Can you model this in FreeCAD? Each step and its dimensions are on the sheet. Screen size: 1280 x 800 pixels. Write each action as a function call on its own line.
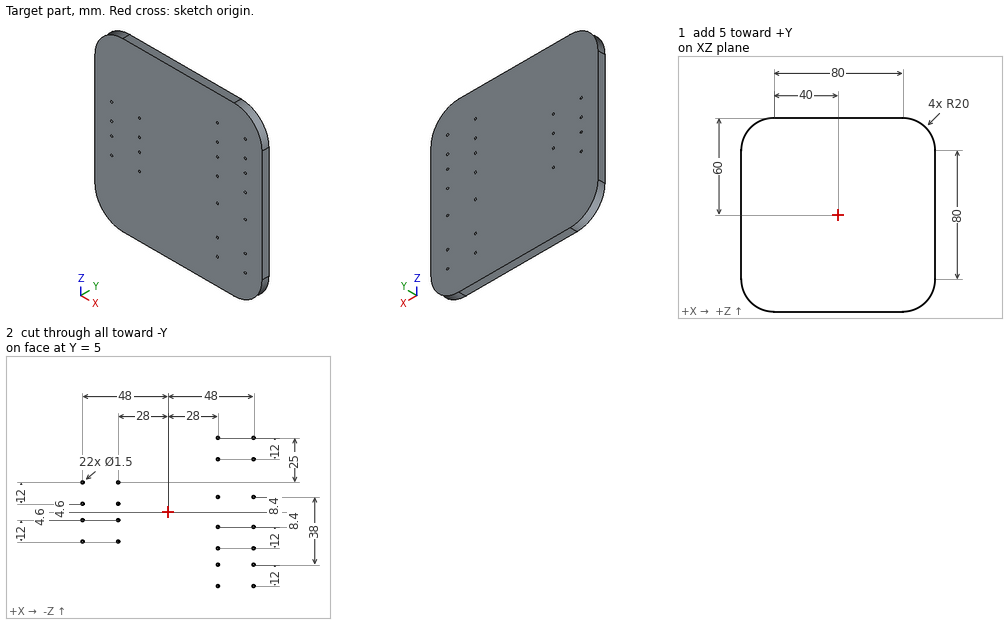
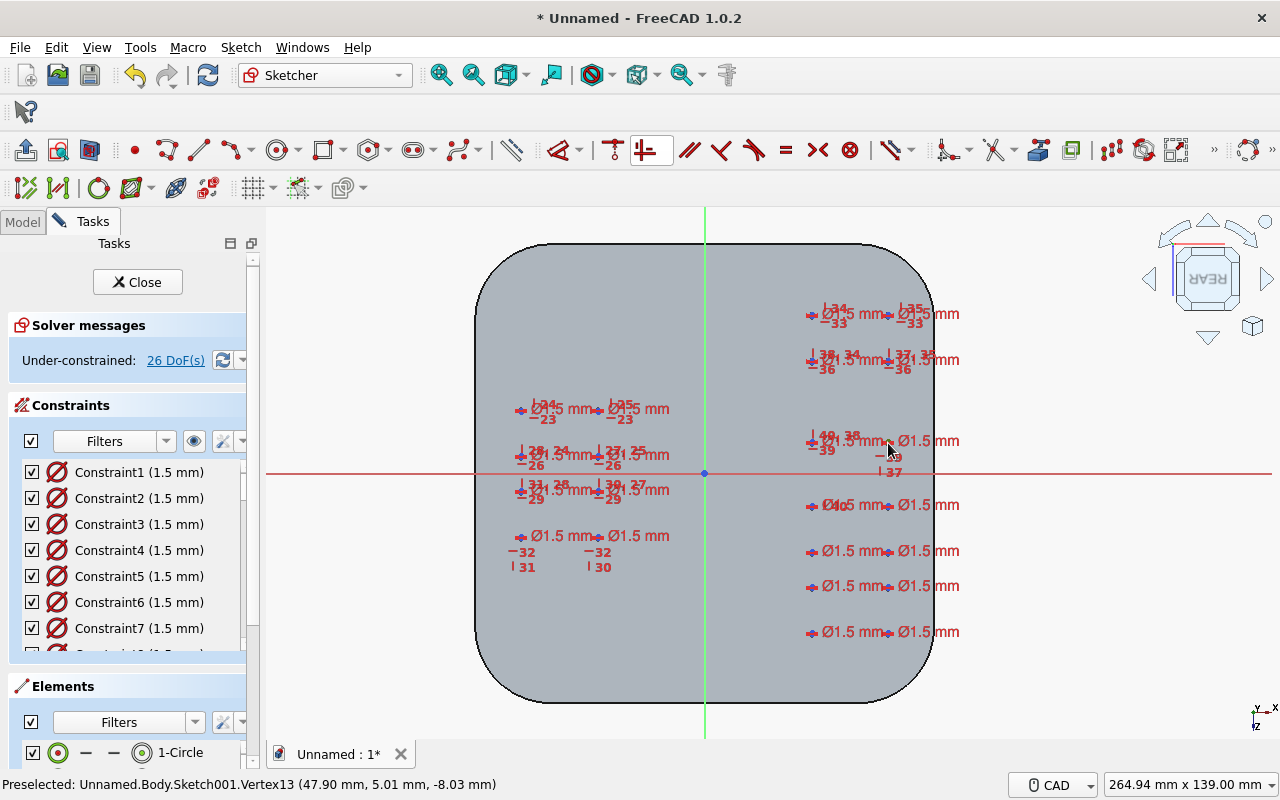
click(888, 507)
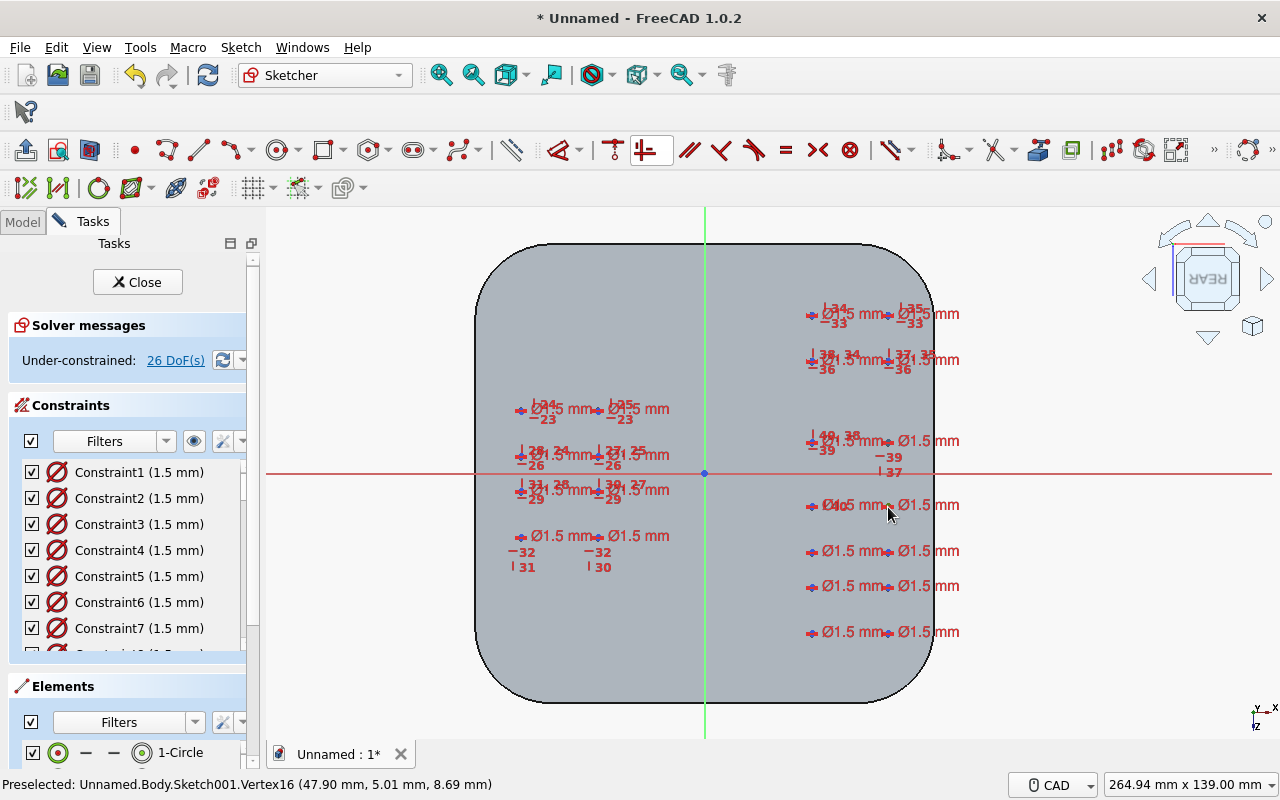
click(668, 150)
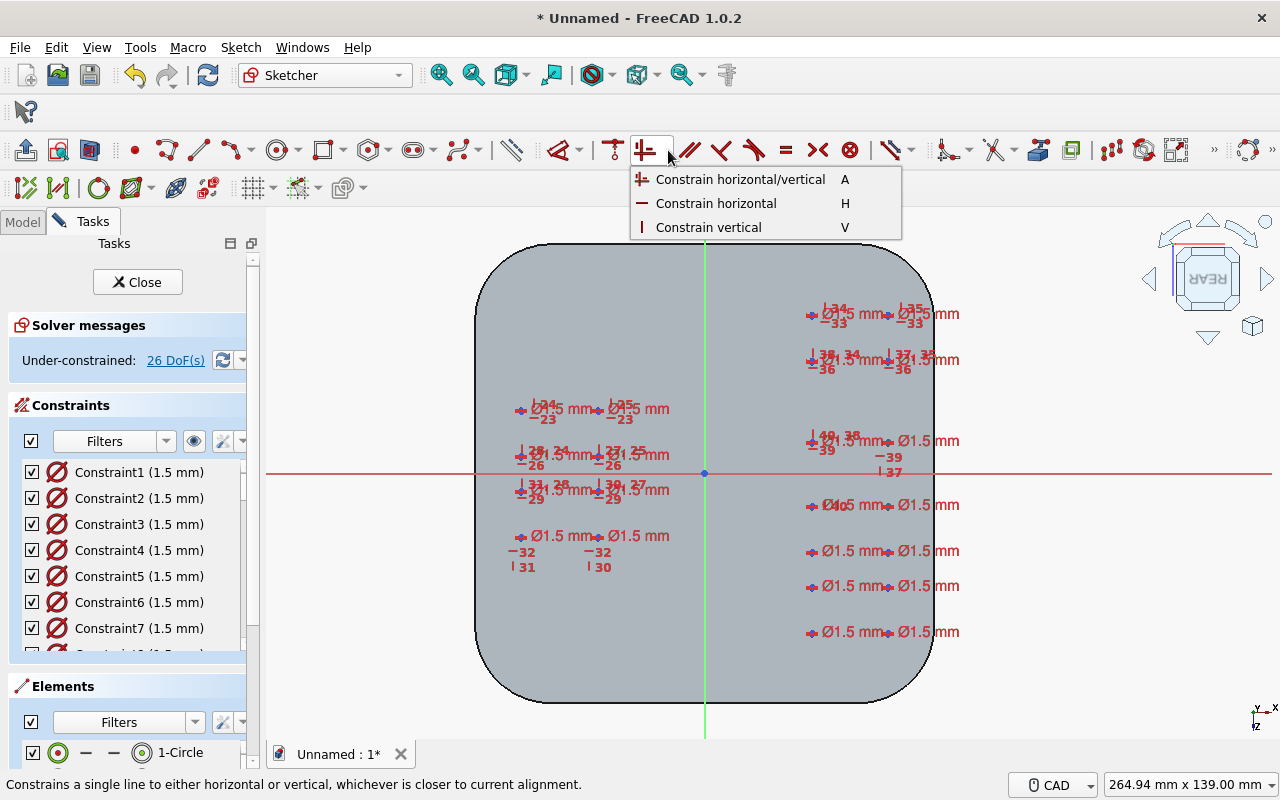
click(766, 227)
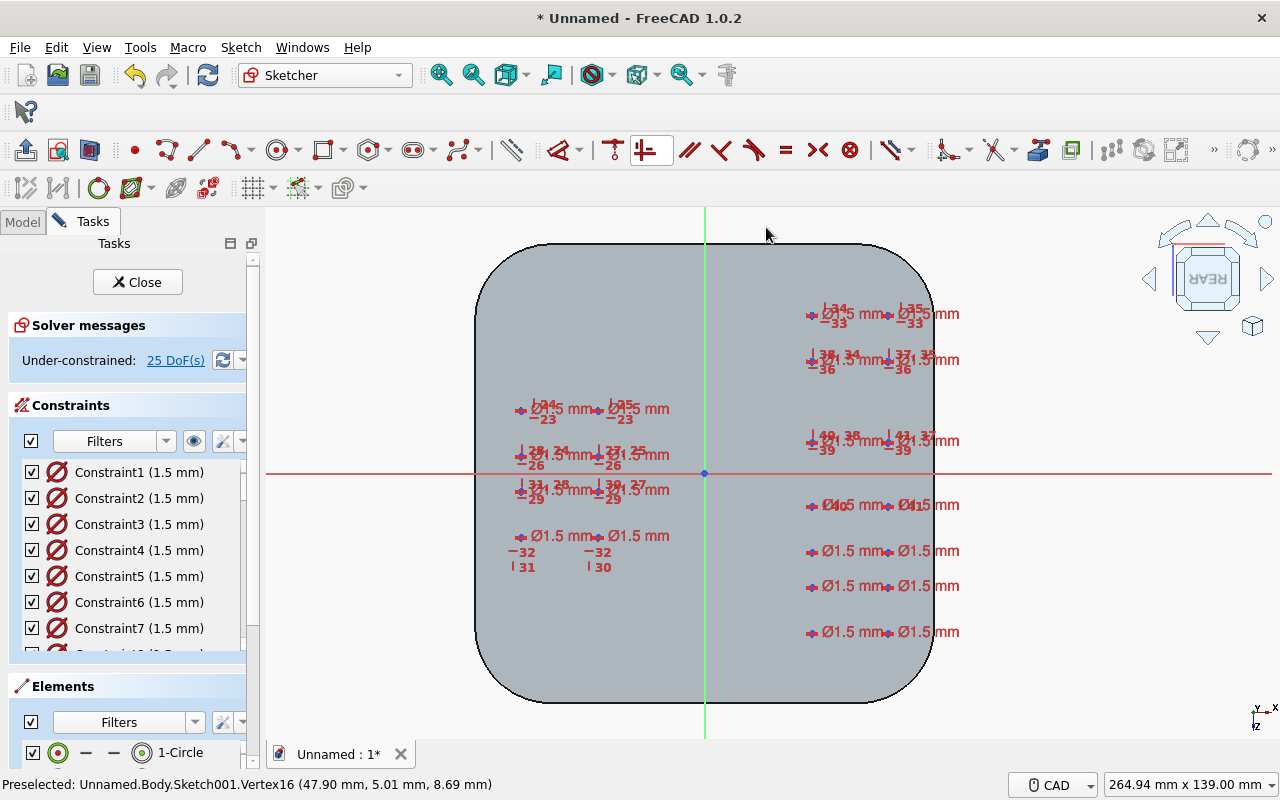
click(812, 507)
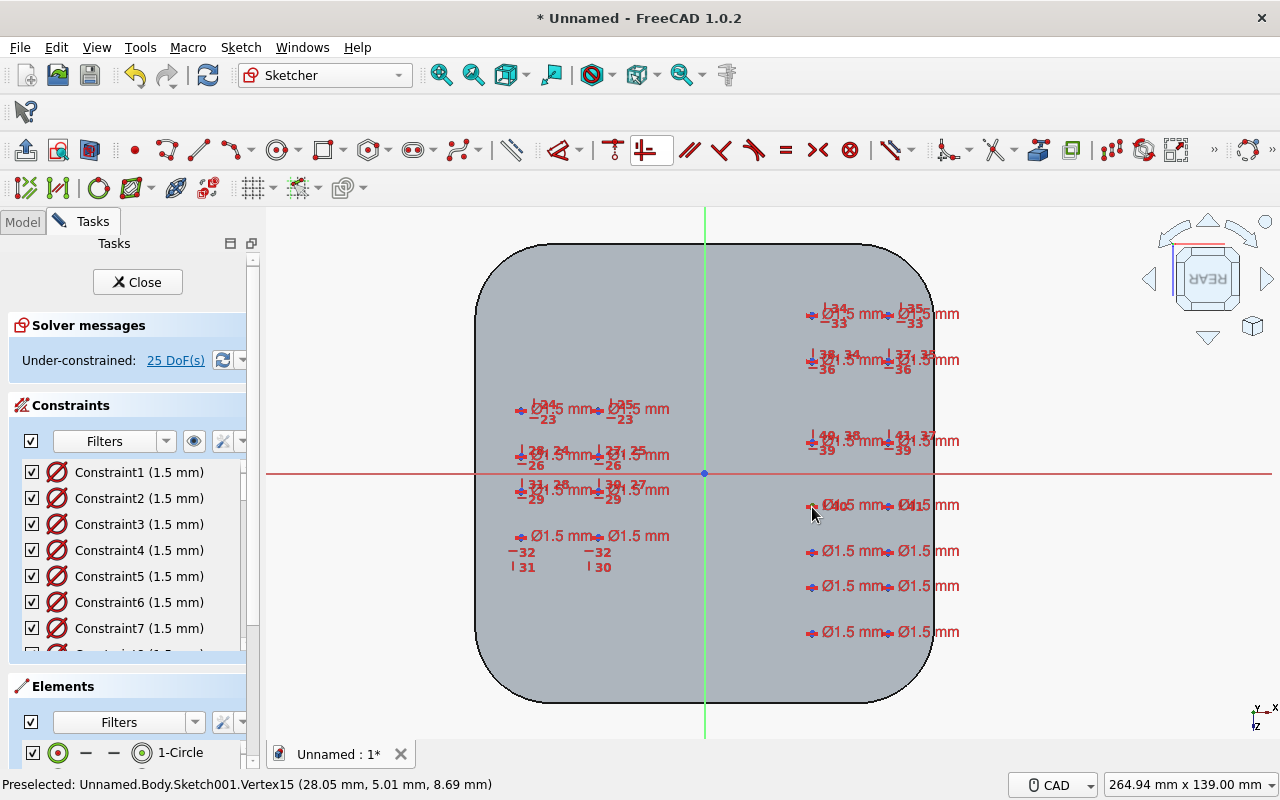
click(888, 507)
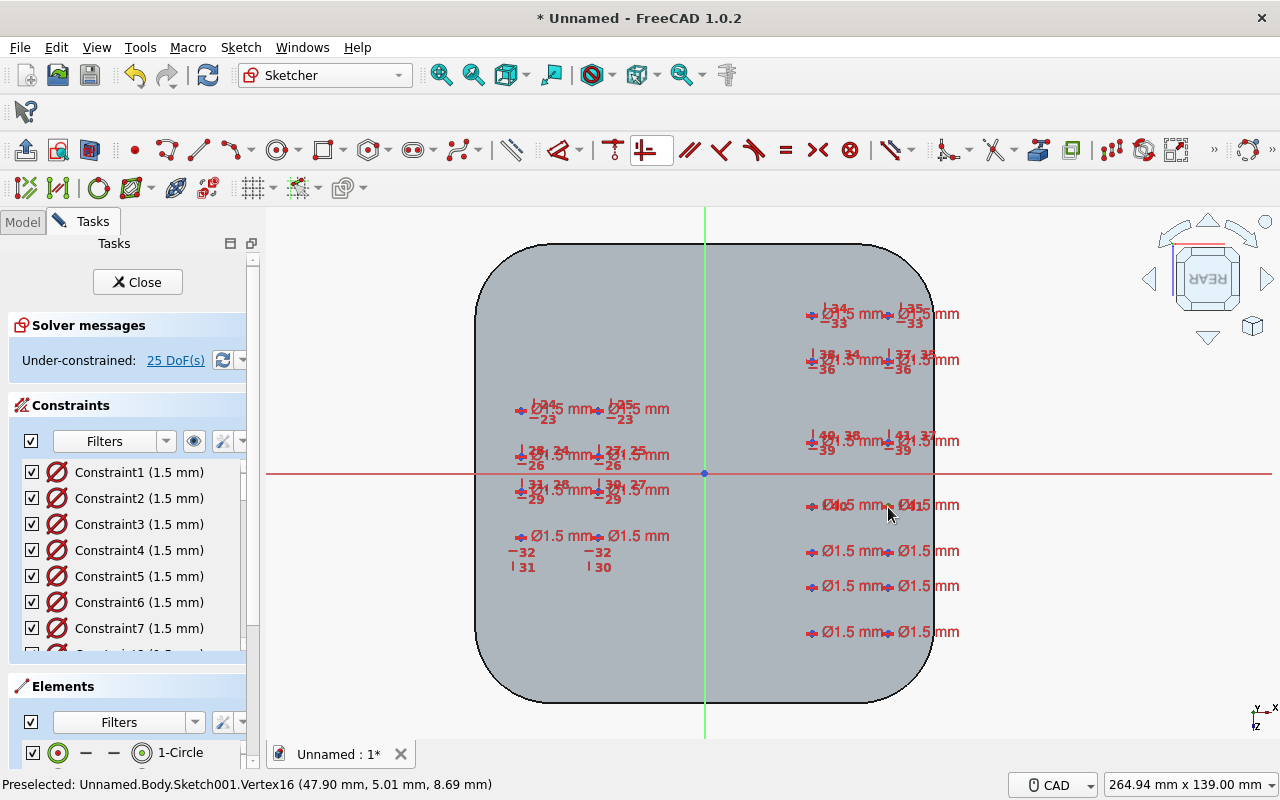
key(h)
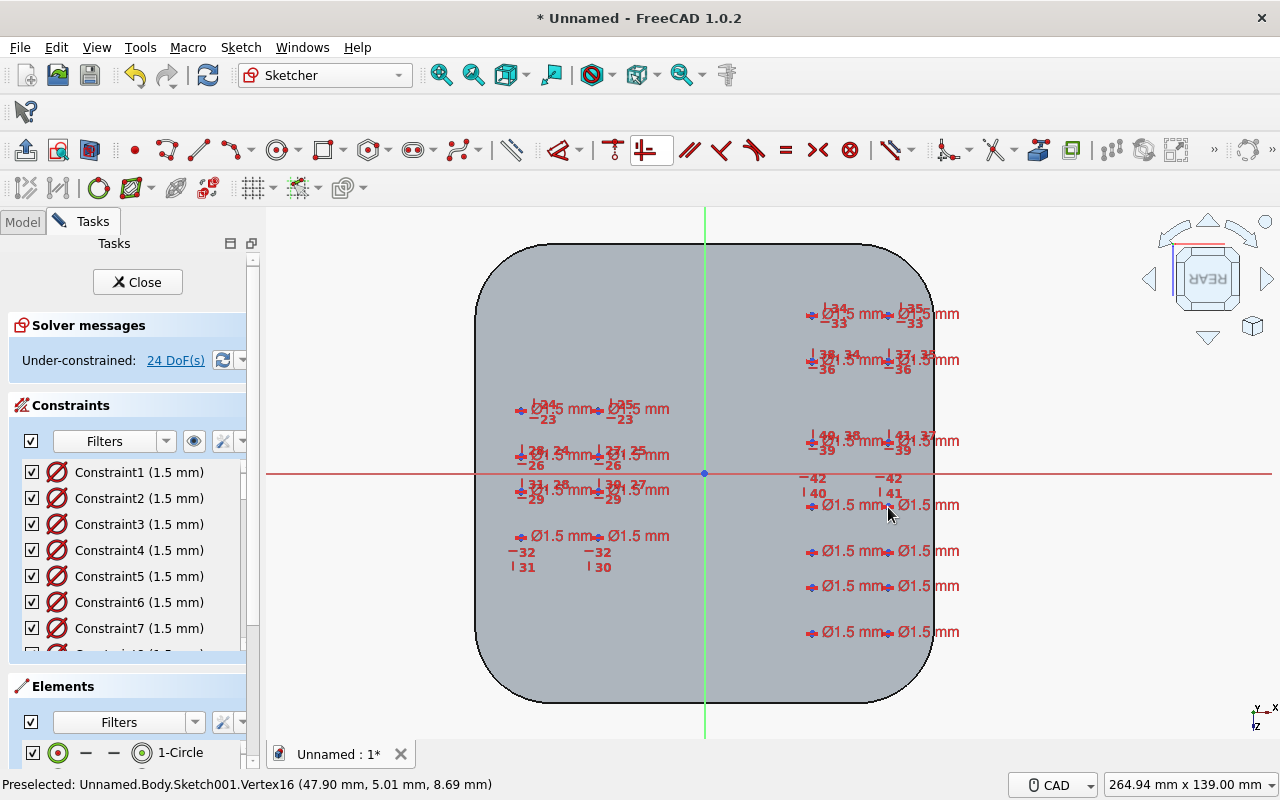
click(812, 507)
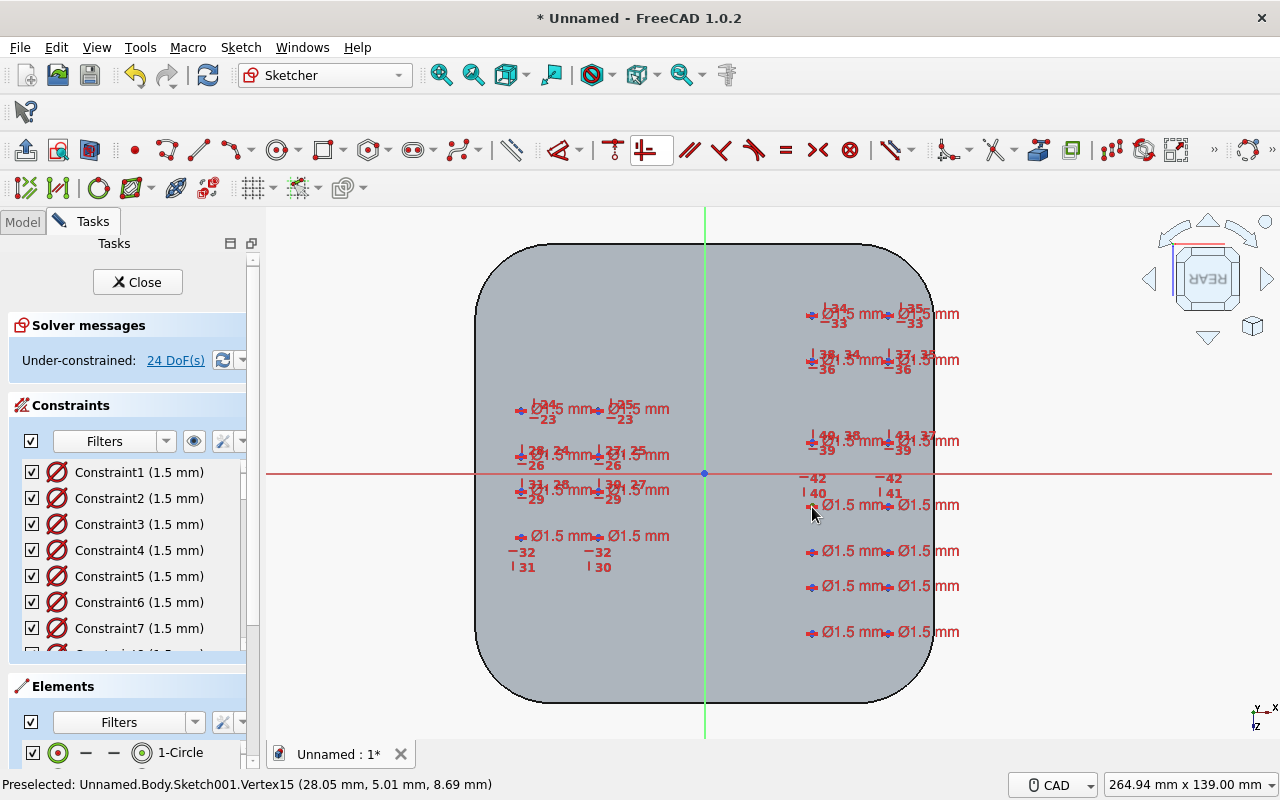
click(812, 553)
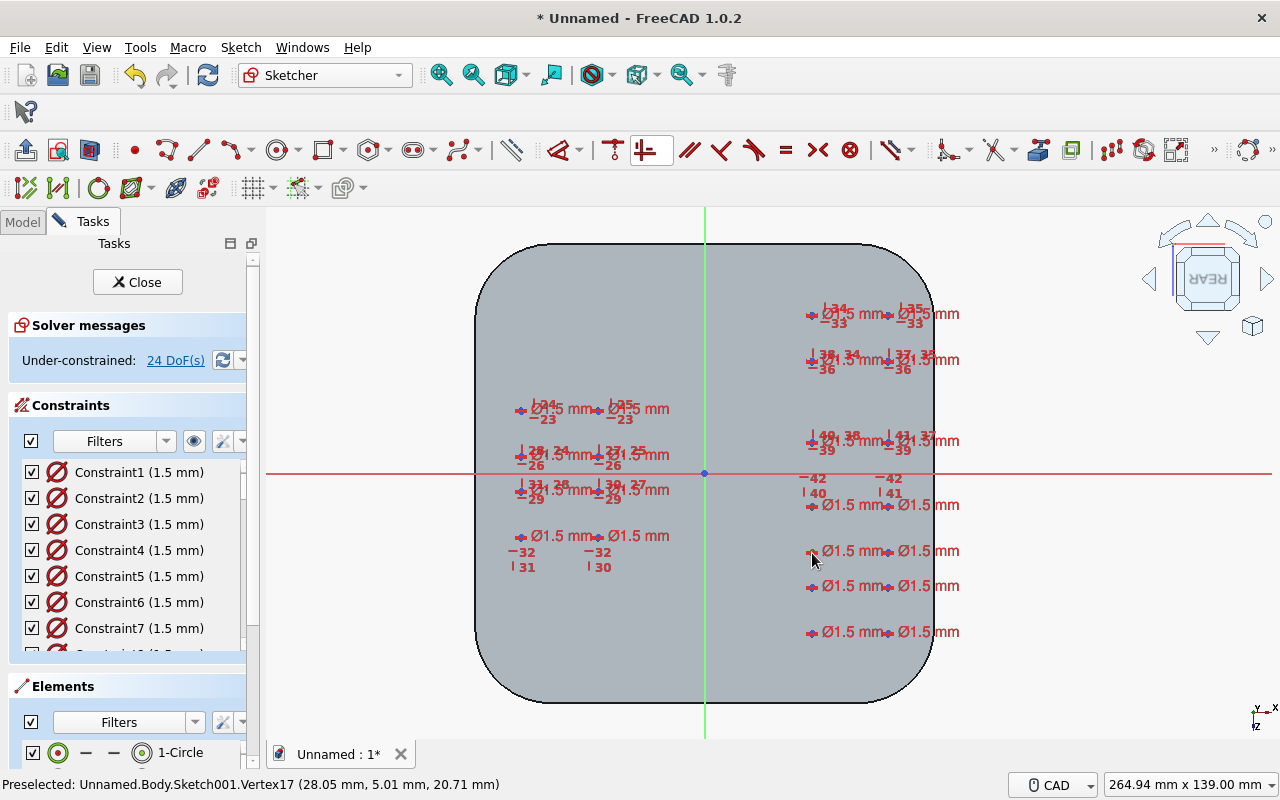
click(668, 150)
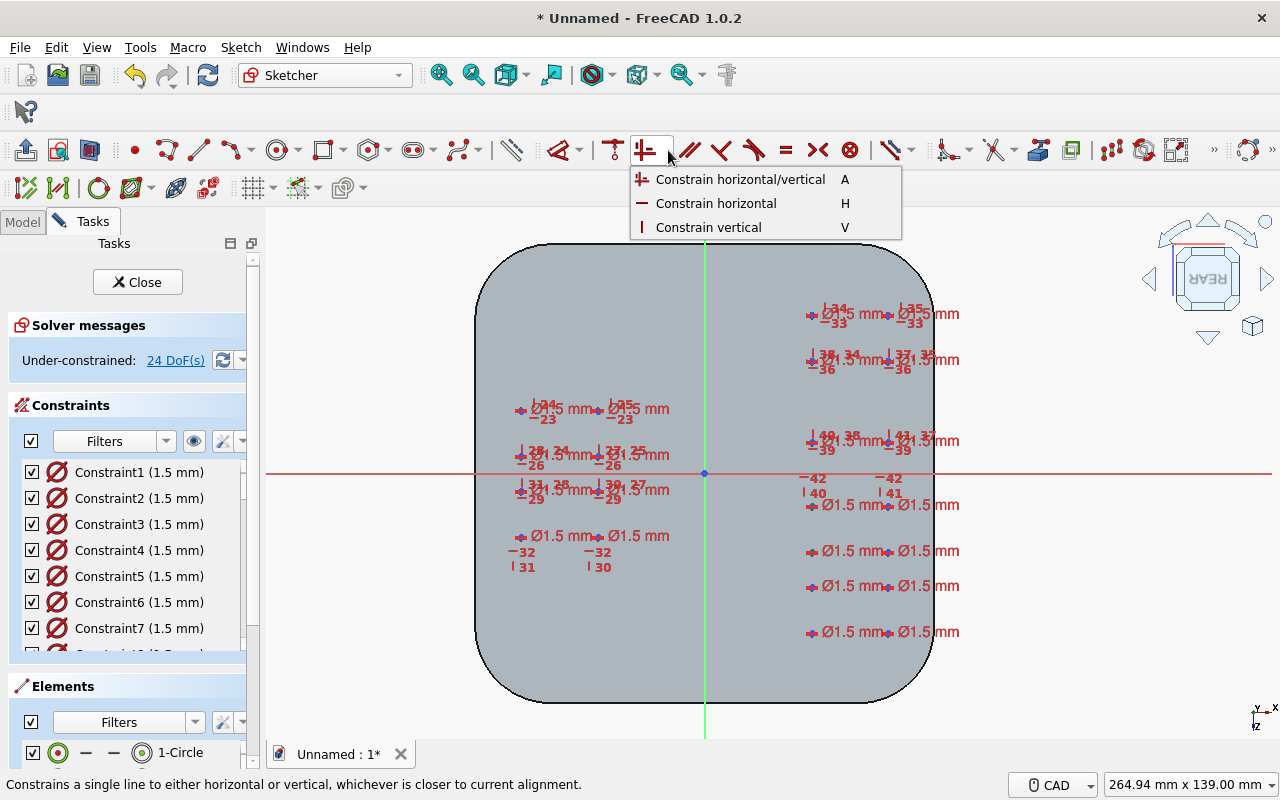
click(766, 227)